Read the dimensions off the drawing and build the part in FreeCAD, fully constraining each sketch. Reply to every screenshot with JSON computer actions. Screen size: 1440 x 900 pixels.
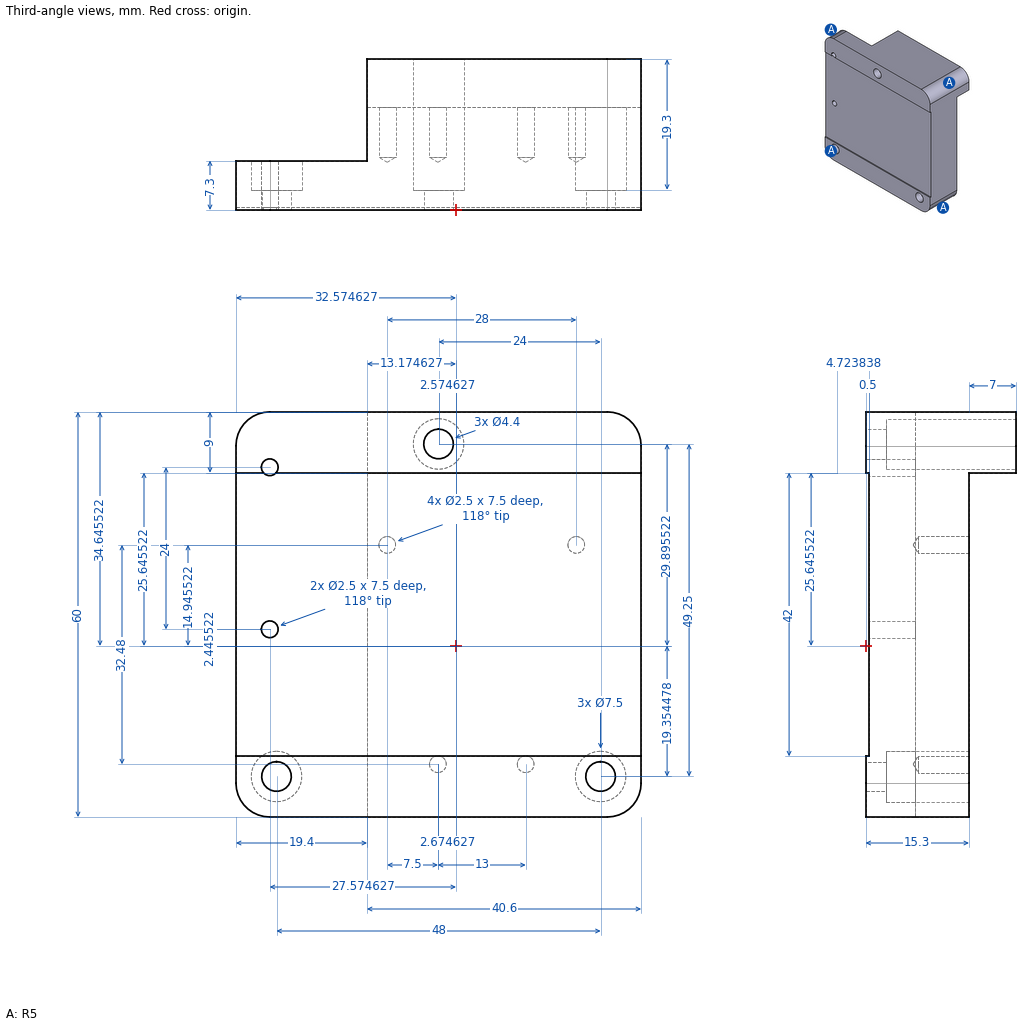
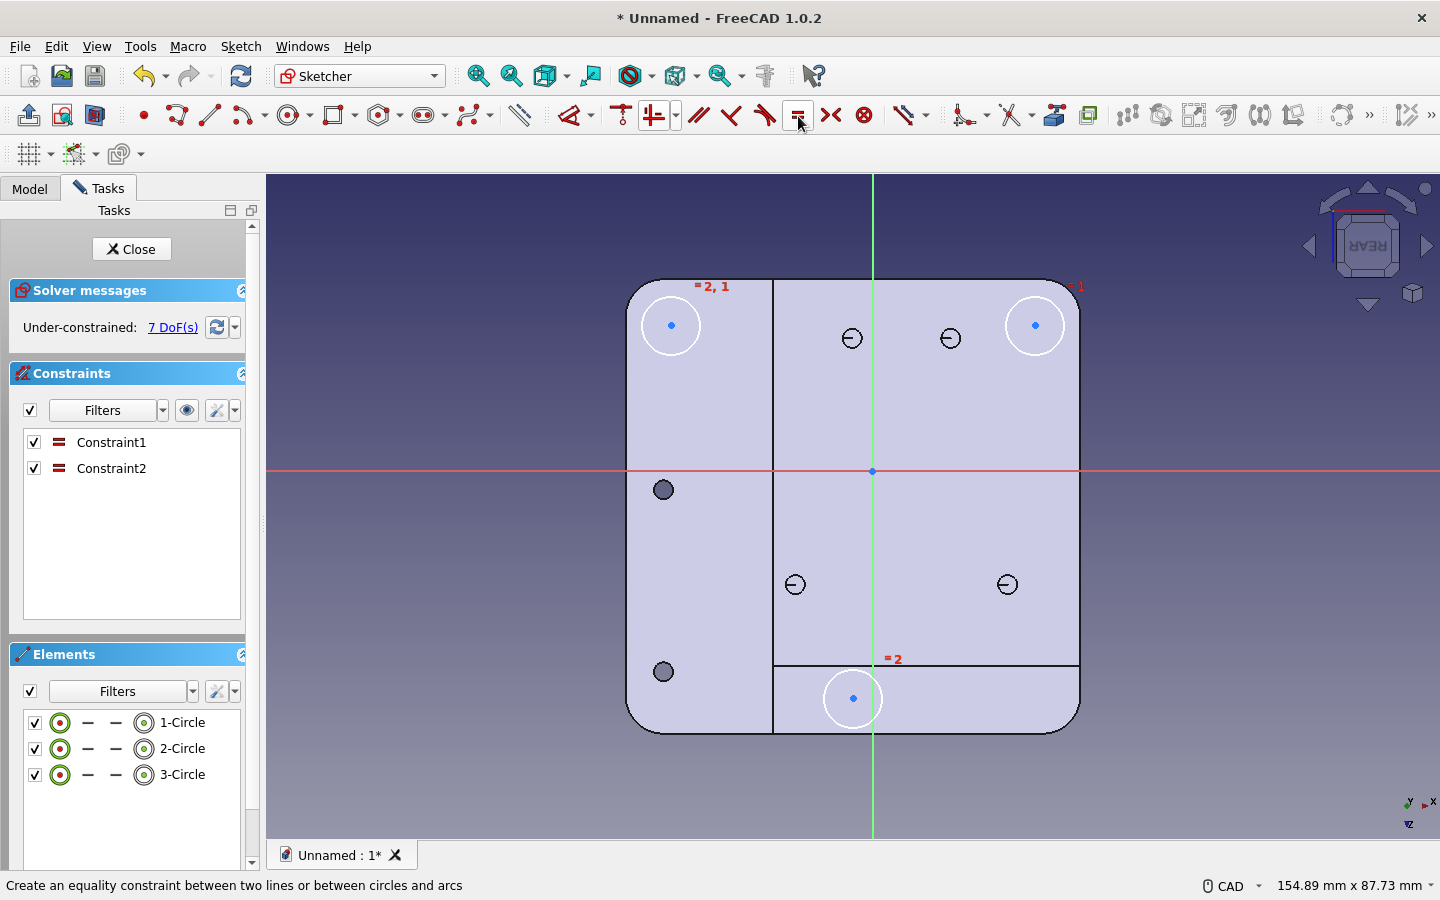
{"action": "left_click", "coordinate": [1035, 326]}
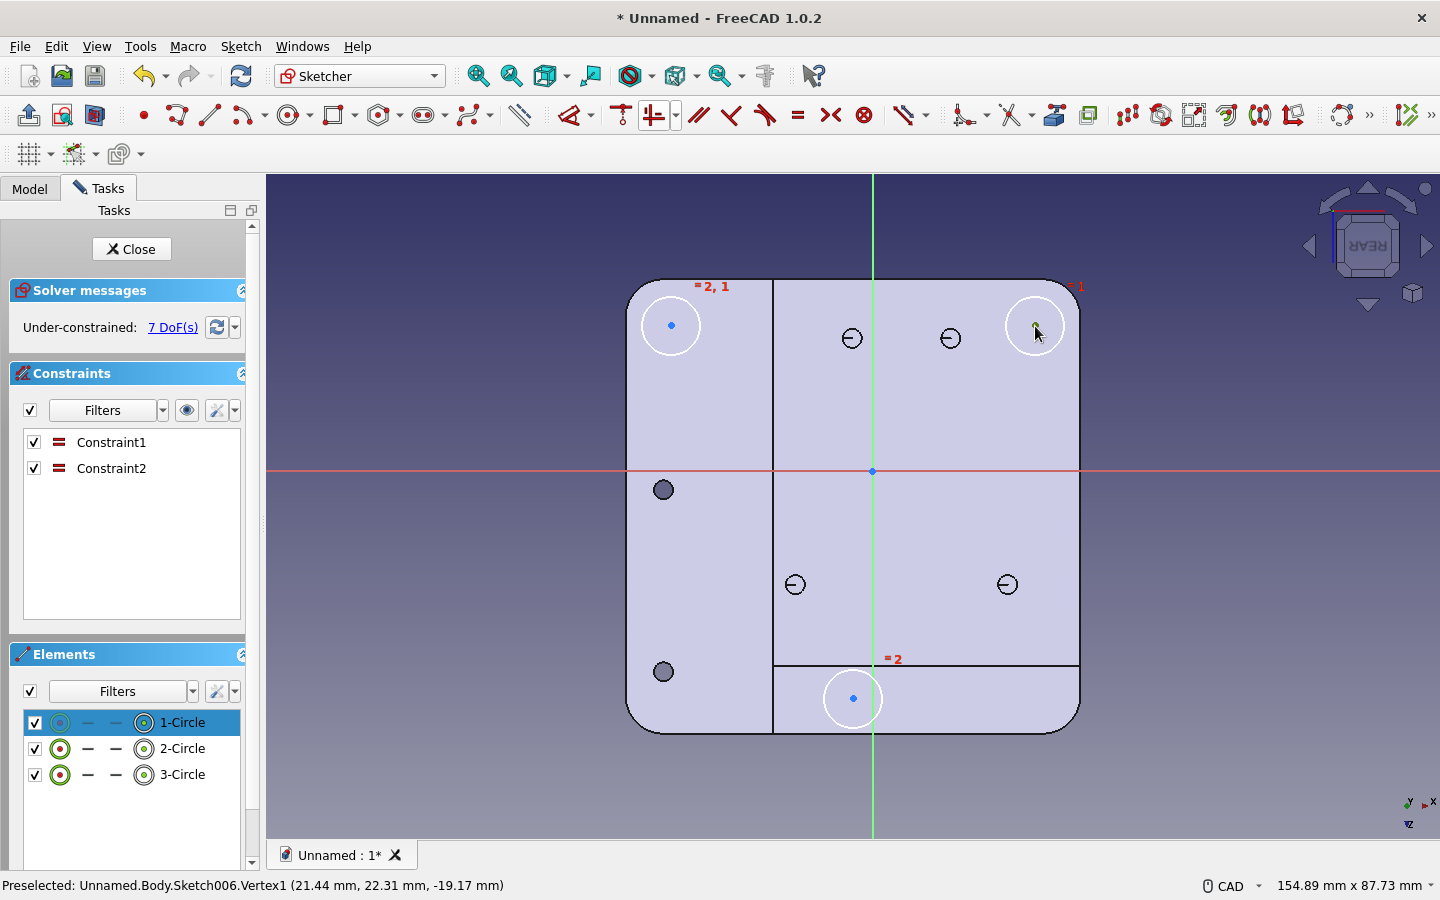
{"action": "left_click", "coordinate": [671, 326]}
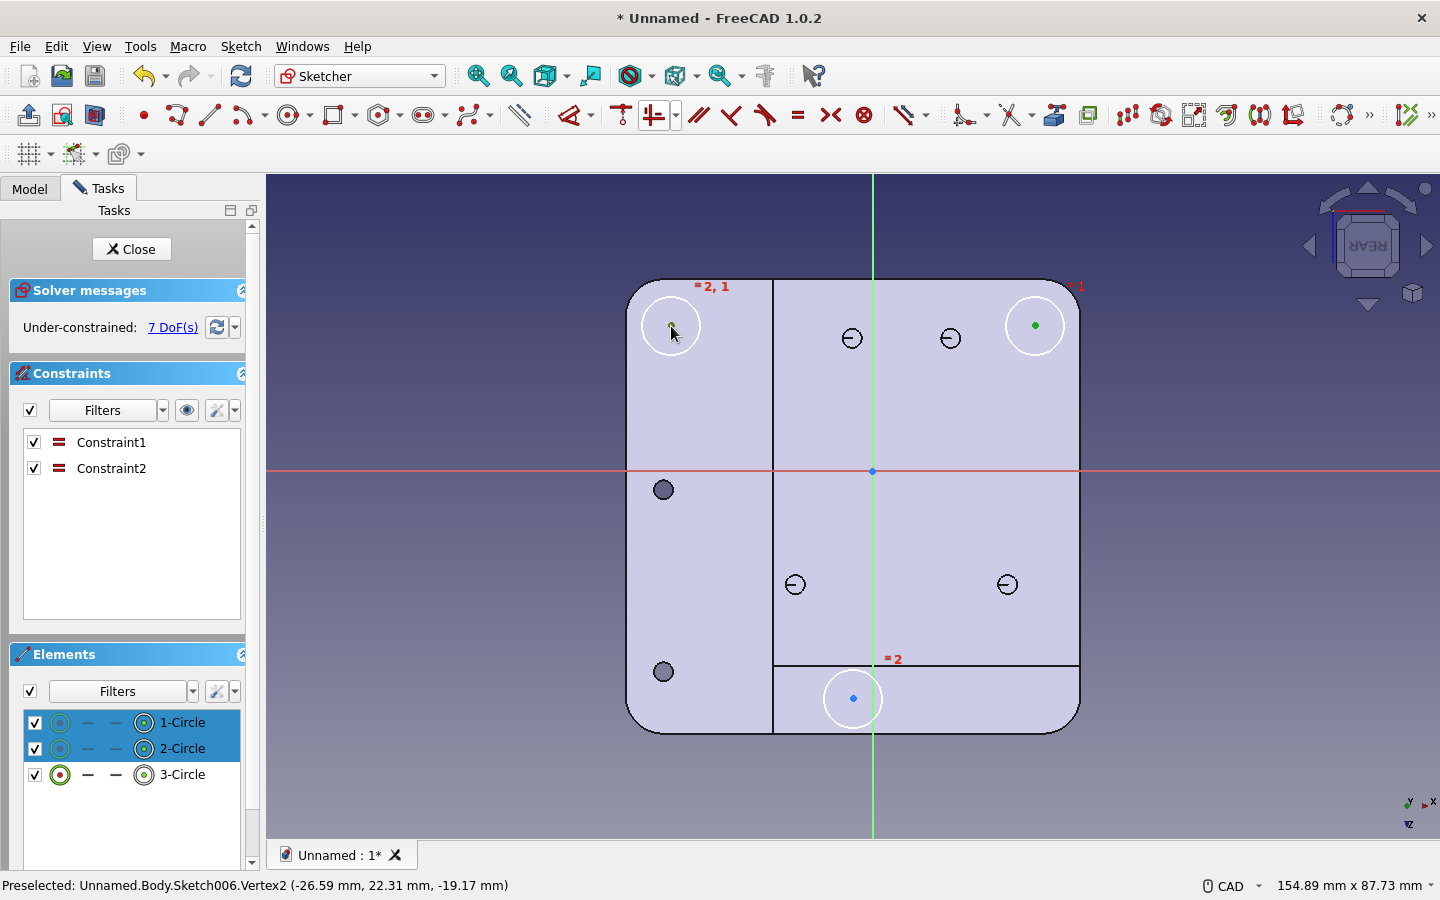
{"action": "left_click", "coordinate": [676, 116]}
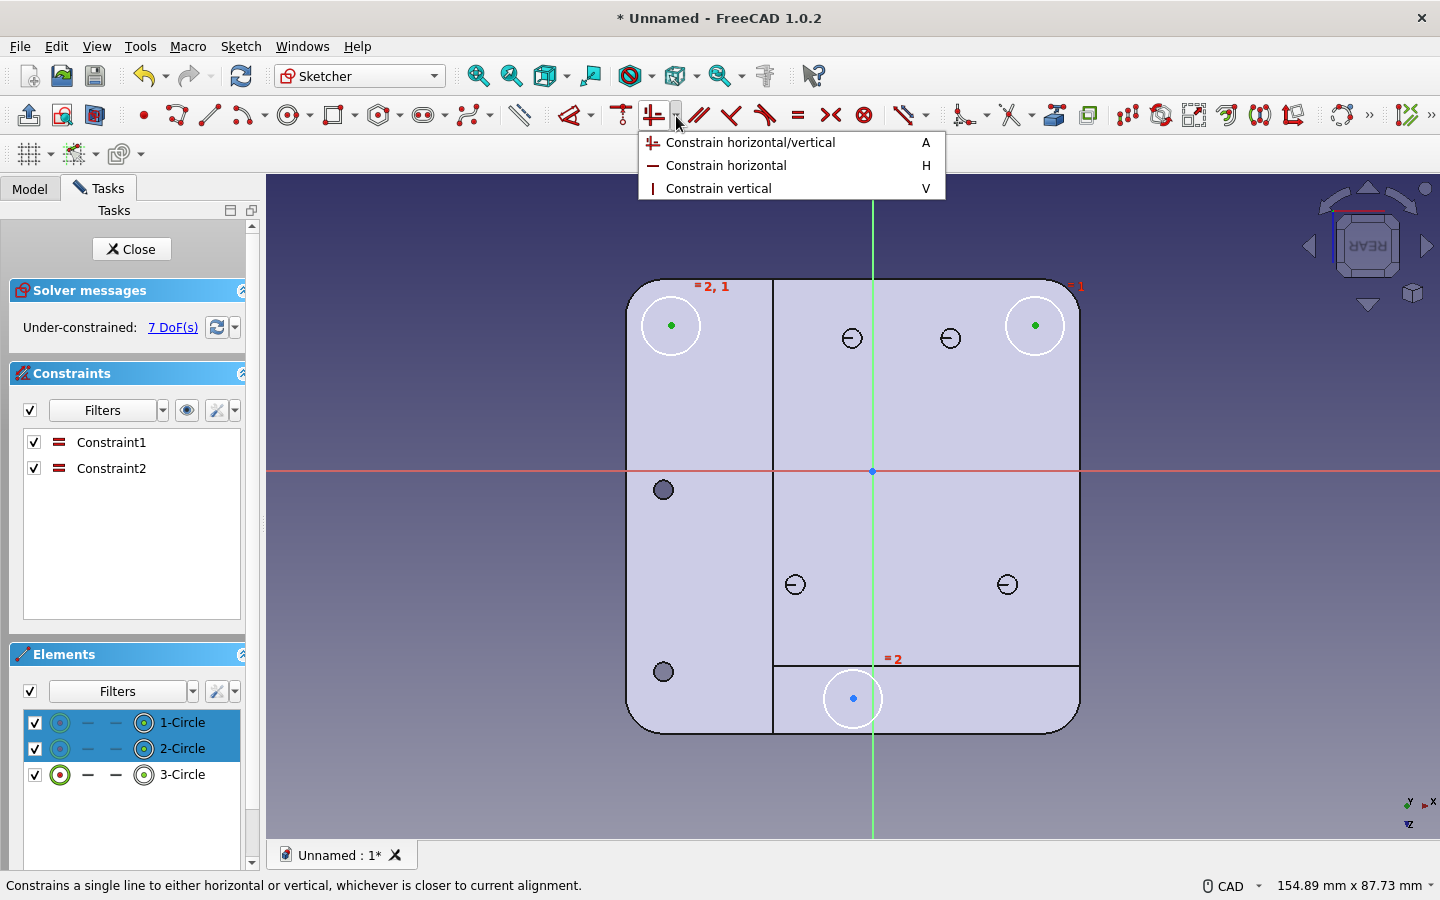
{"action": "left_click", "coordinate": [792, 166]}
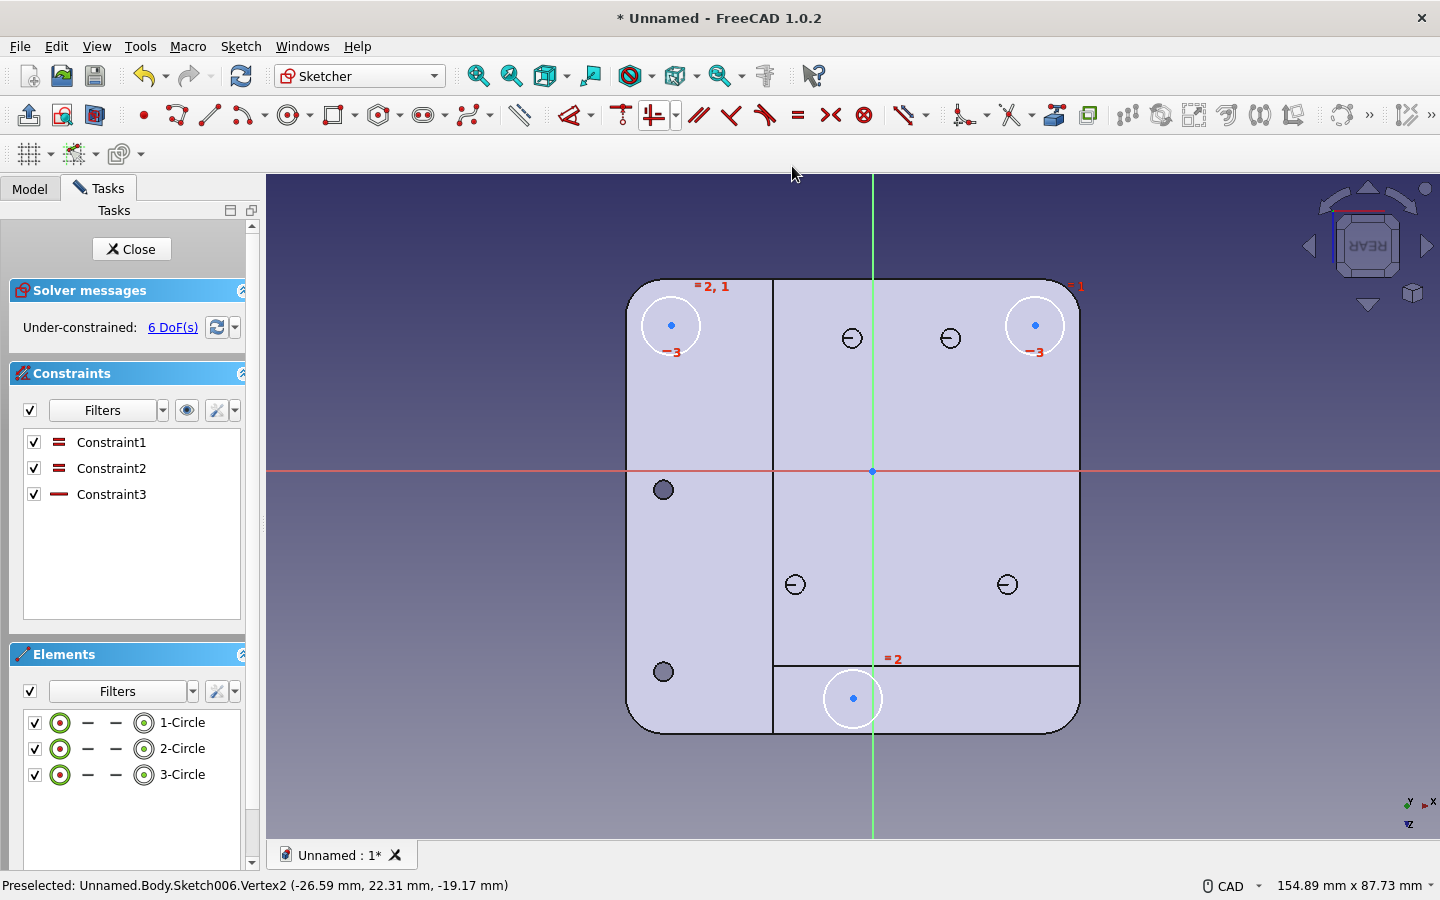
{"action": "key", "text": "d"}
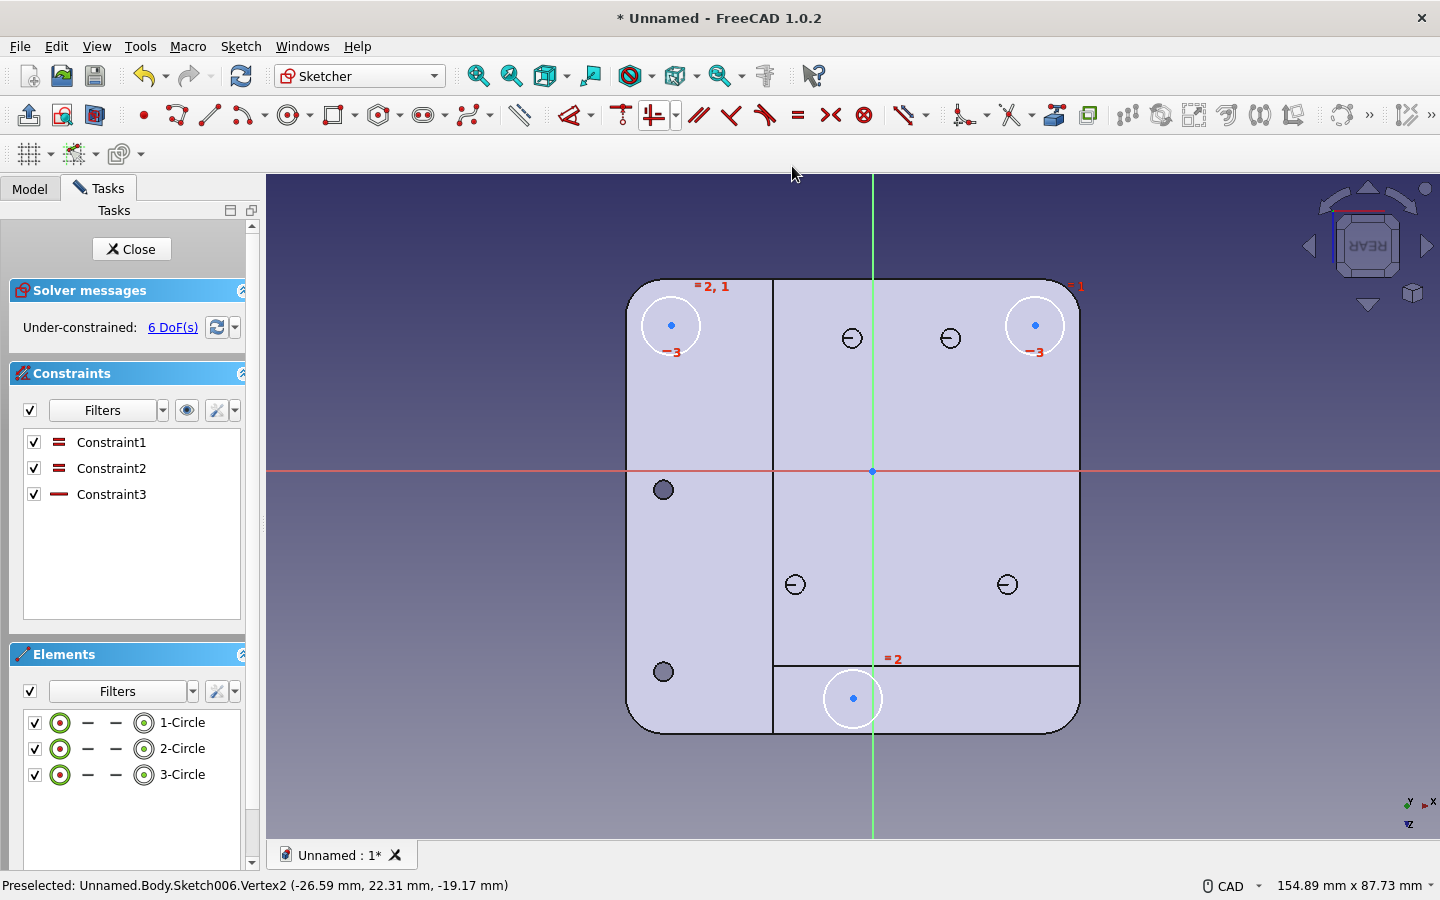
{"action": "left_click", "coordinate": [1055, 305]}
{"action": "left_click", "coordinate": [1077, 282]}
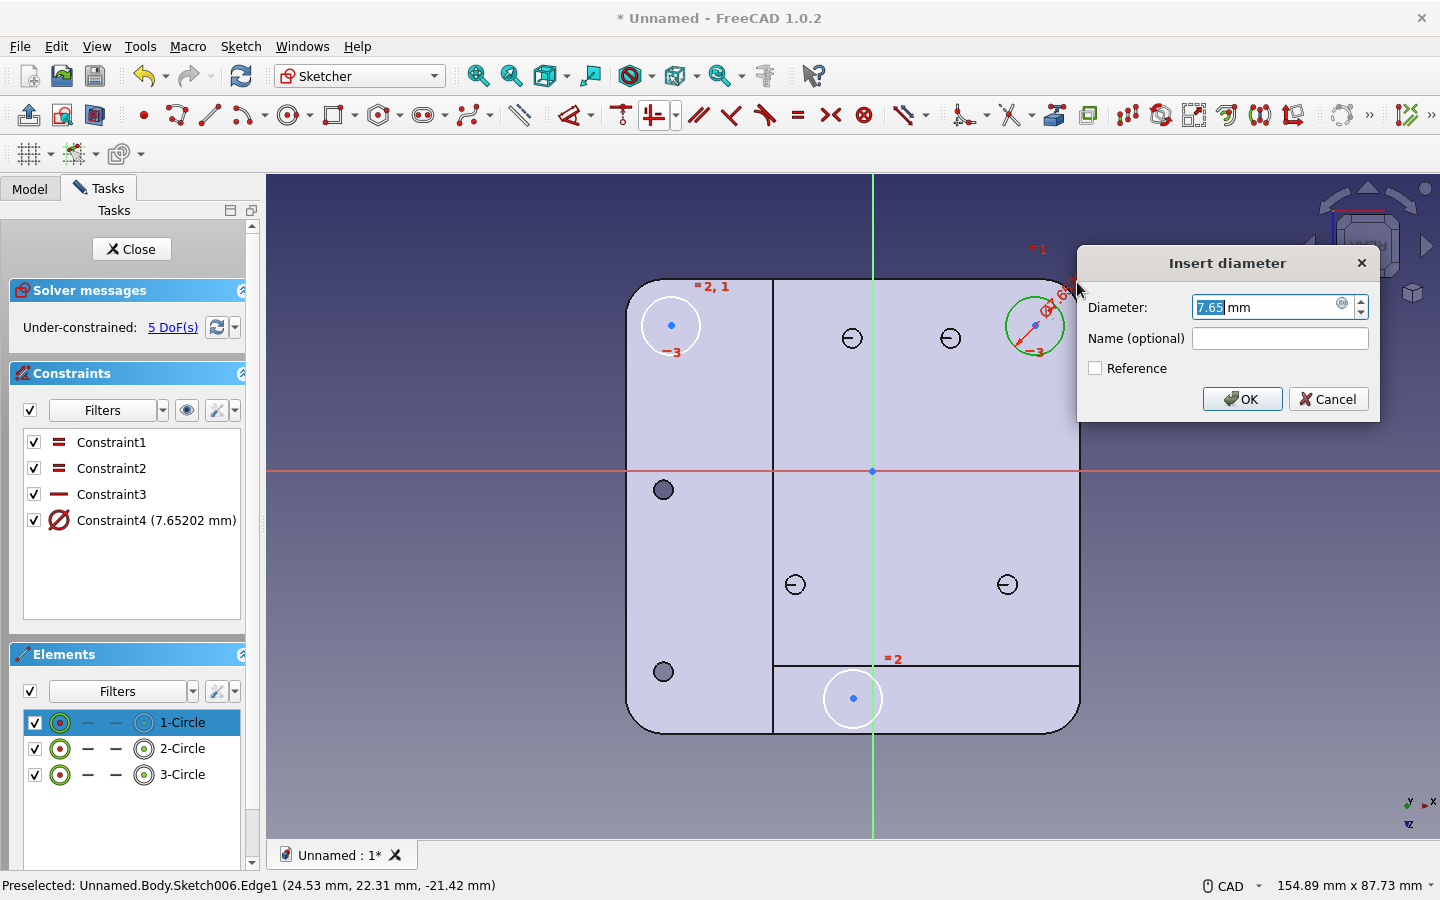
{"action": "type", "text": "7.5"}
{"action": "key", "text": "Return"}